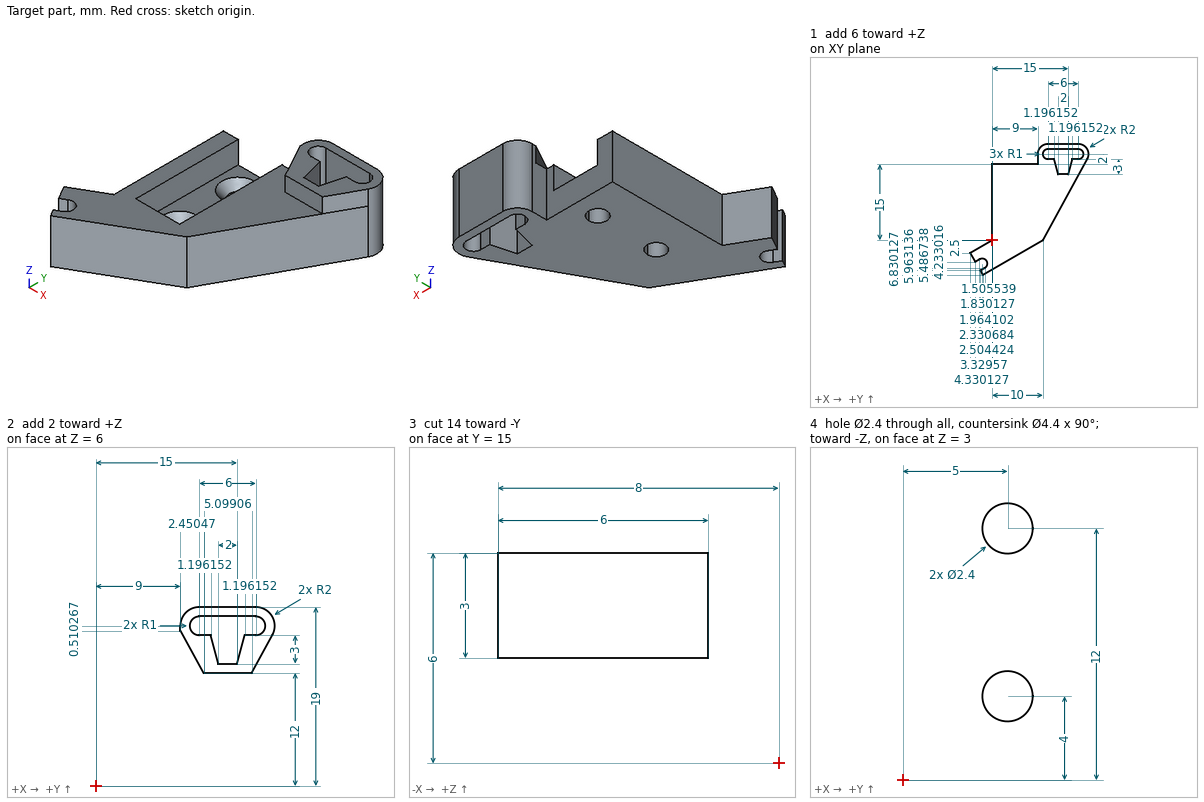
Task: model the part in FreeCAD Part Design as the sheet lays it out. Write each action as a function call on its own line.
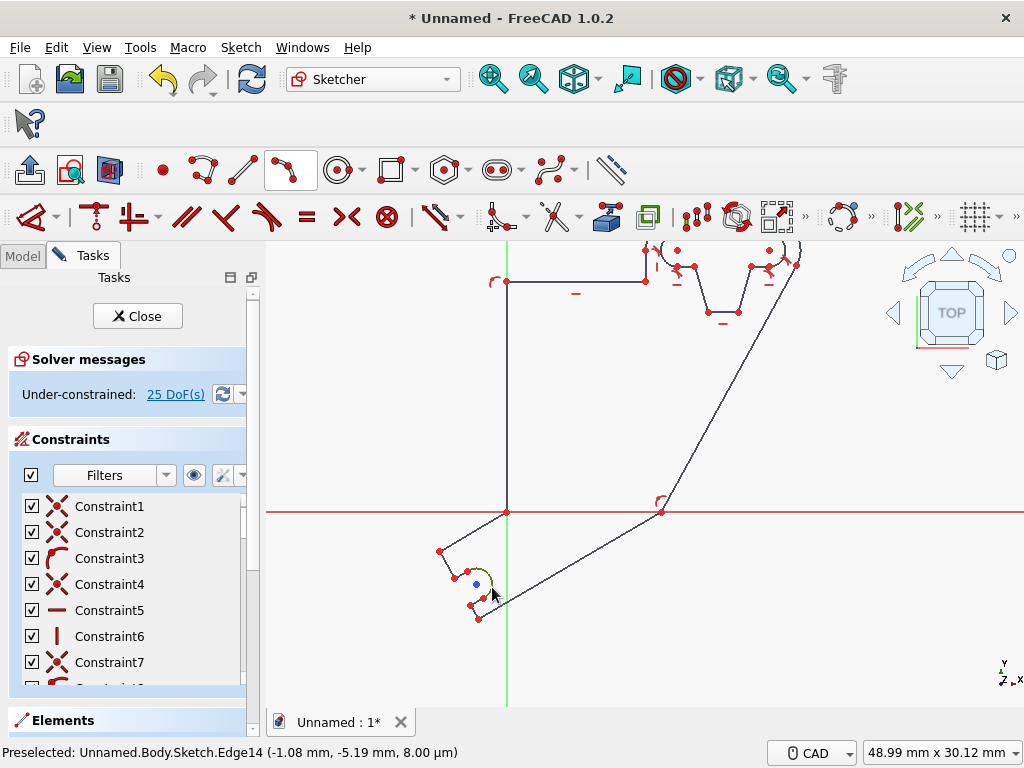
scroll(492, 588, down, 2)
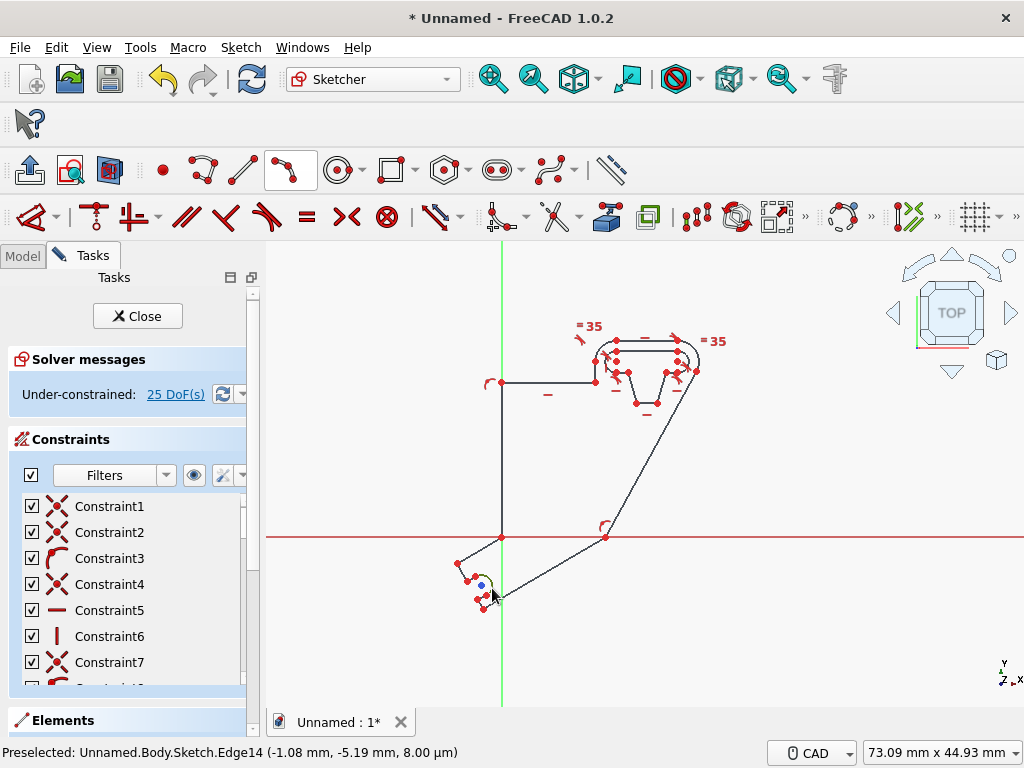
scroll(687, 368, up, 2)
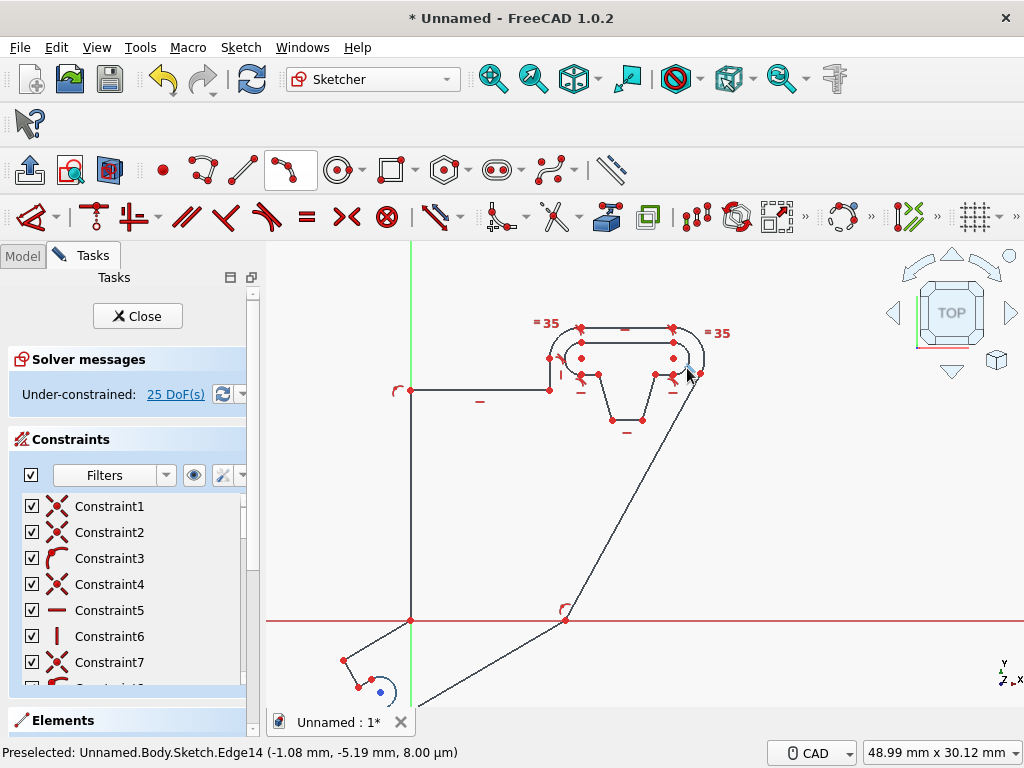
click(686, 349)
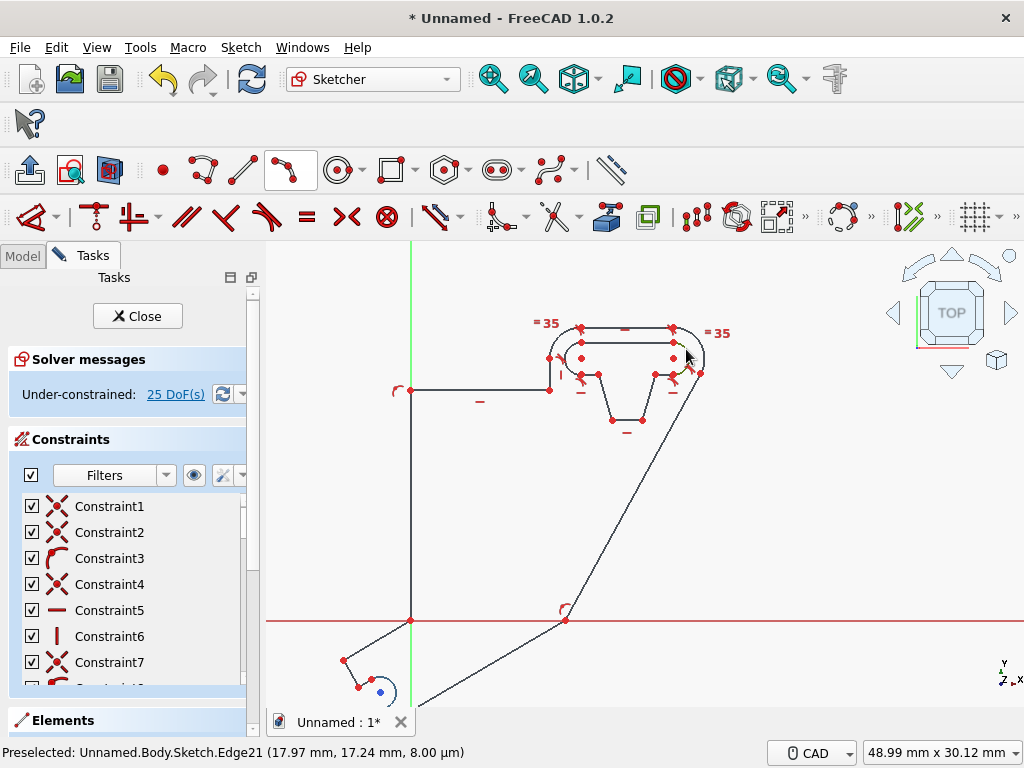
click(308, 218)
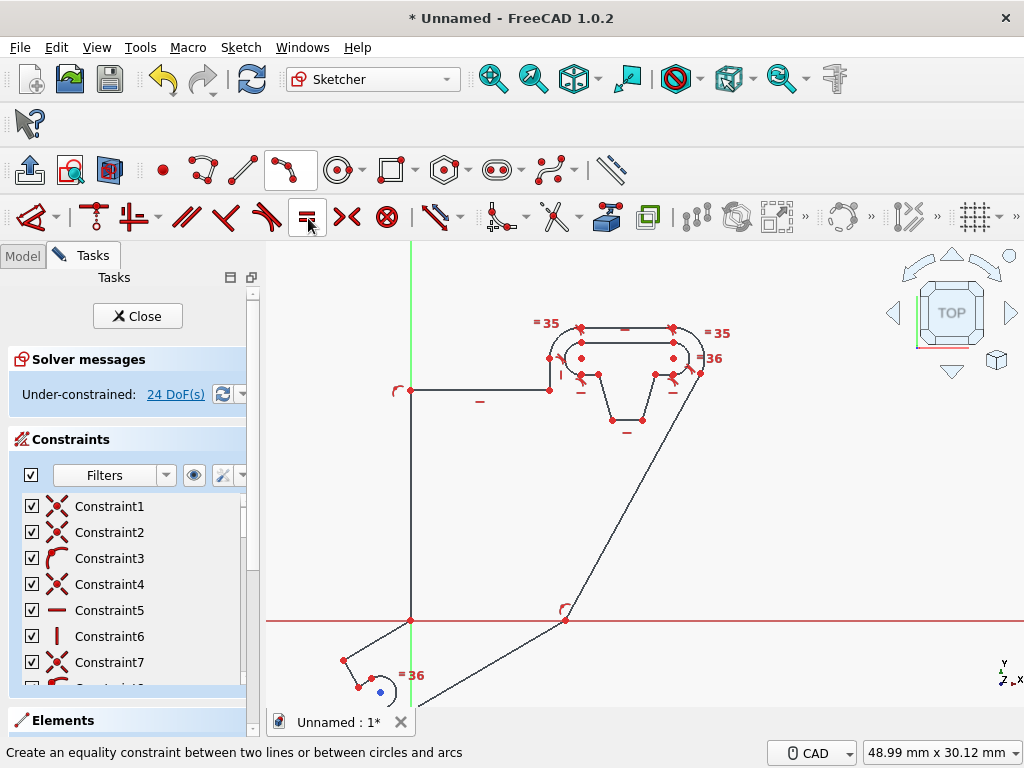
key(d)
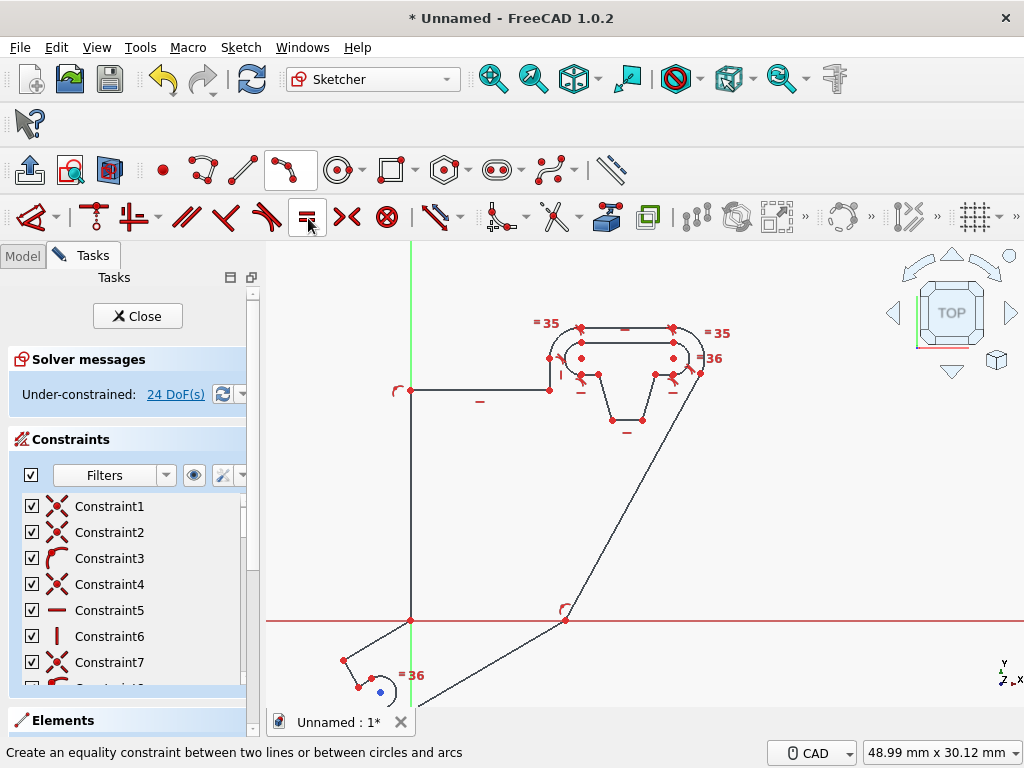
scroll(704, 355, up, 2)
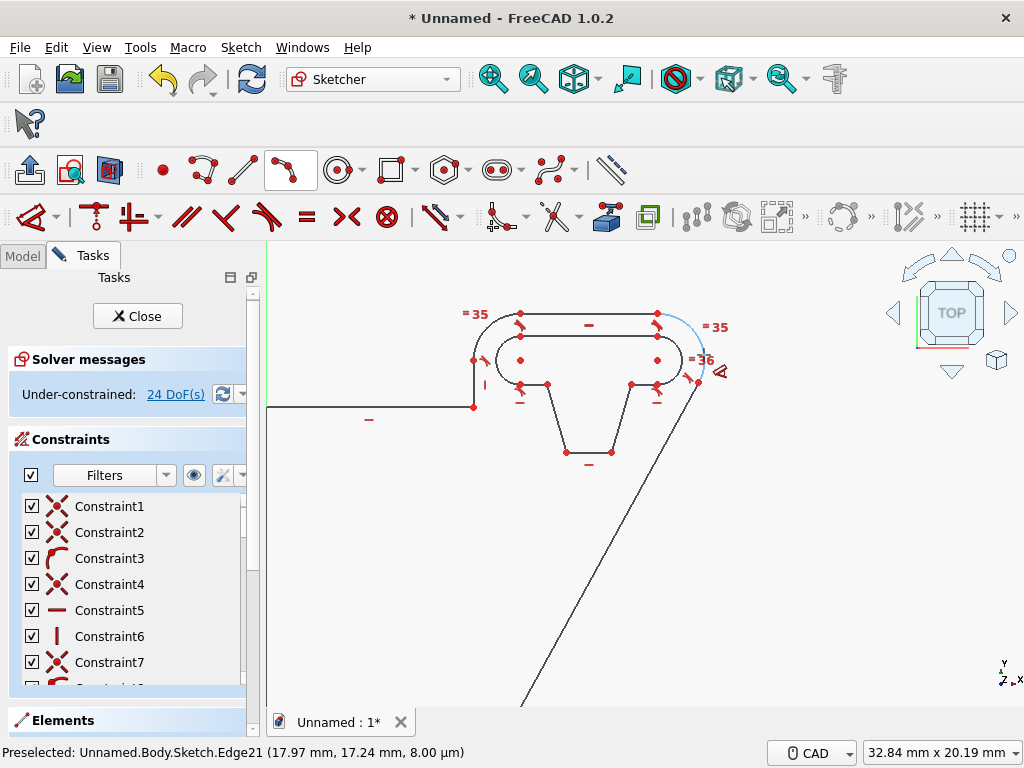
click(704, 355)
click(736, 351)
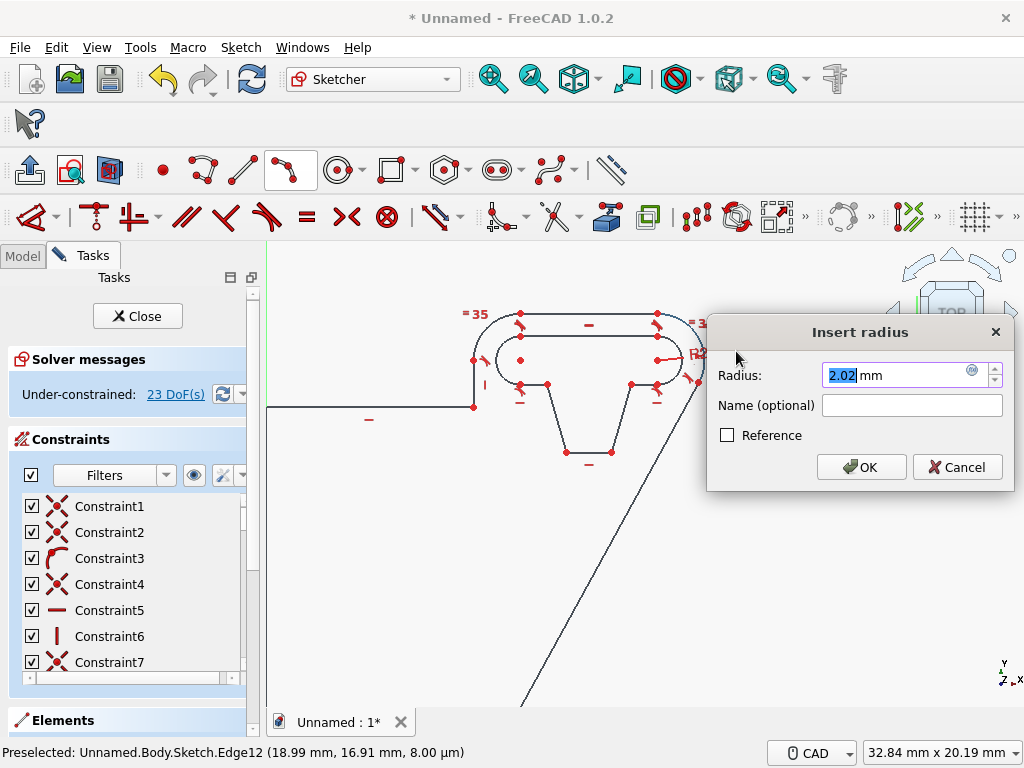
text(2)
key(Return)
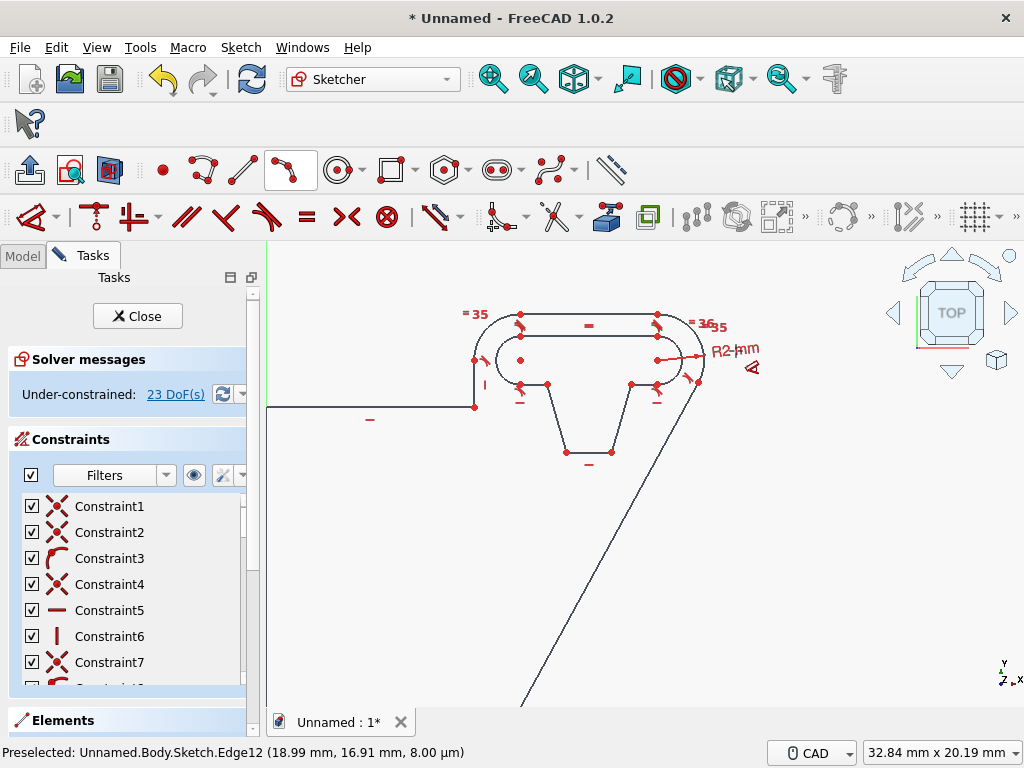
scroll(694, 363, down, 4)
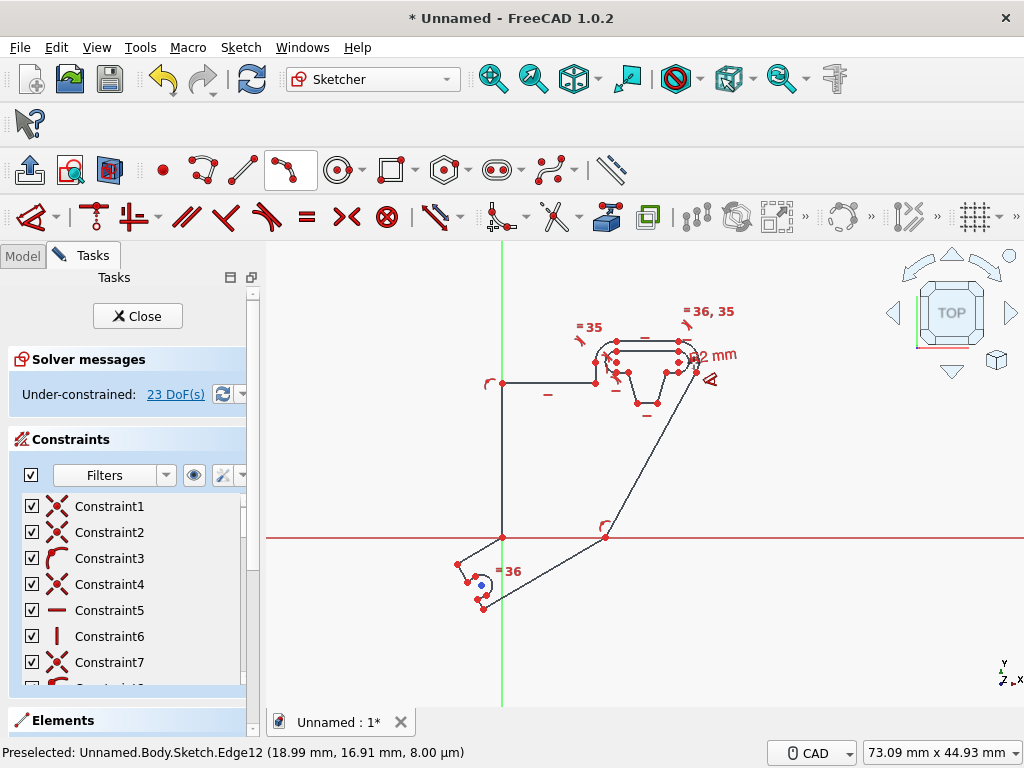
scroll(492, 587, up, 7)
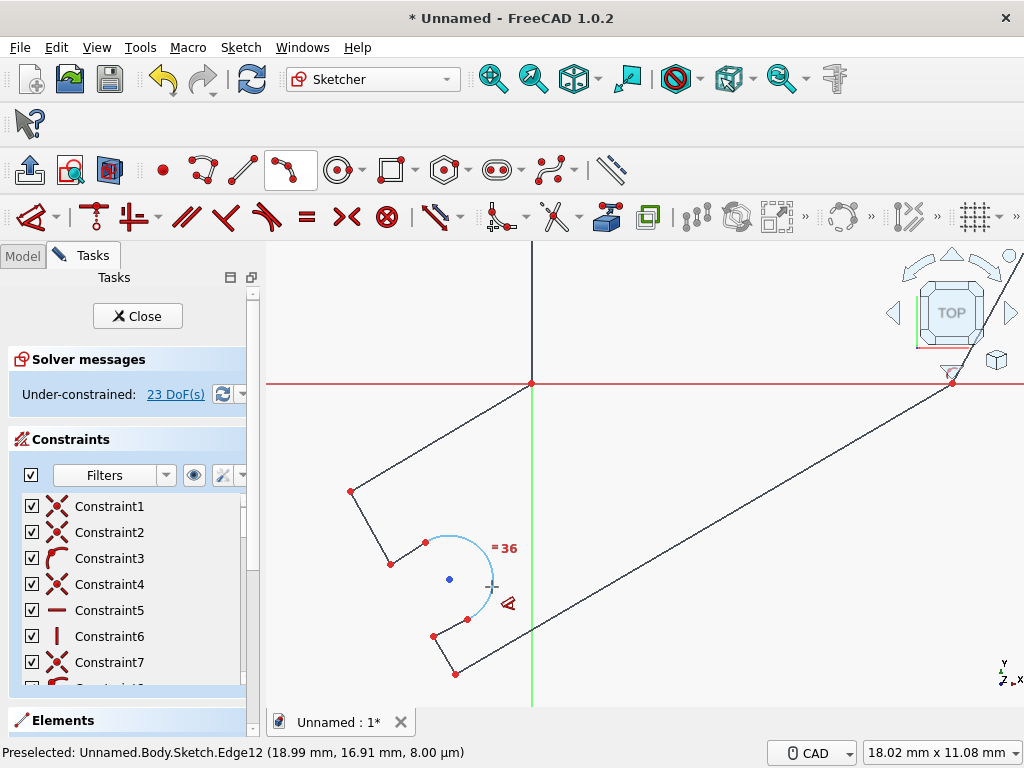
click(493, 586)
click(510, 626)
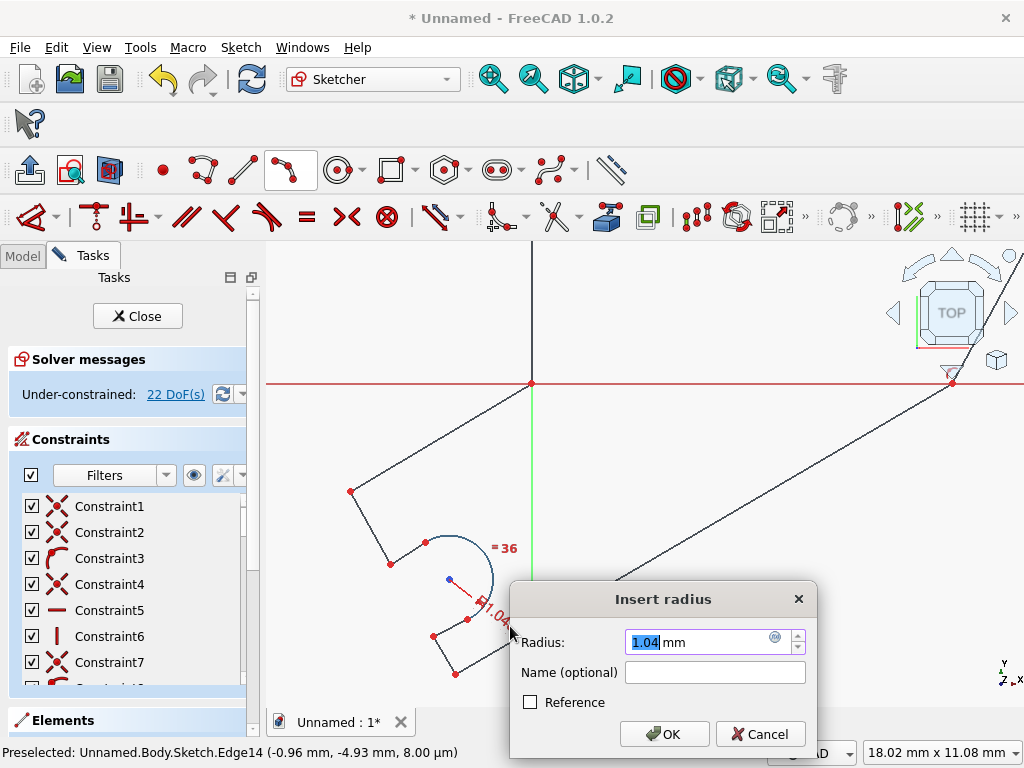
text(1)
key(Return)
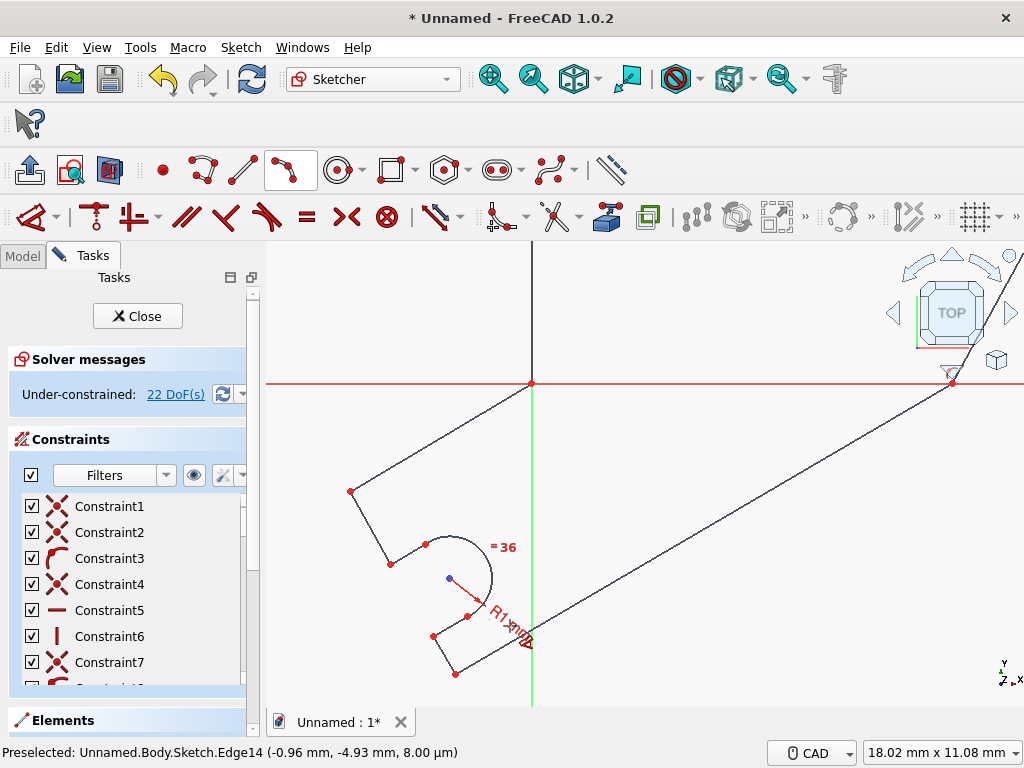
scroll(492, 587, down, 7)